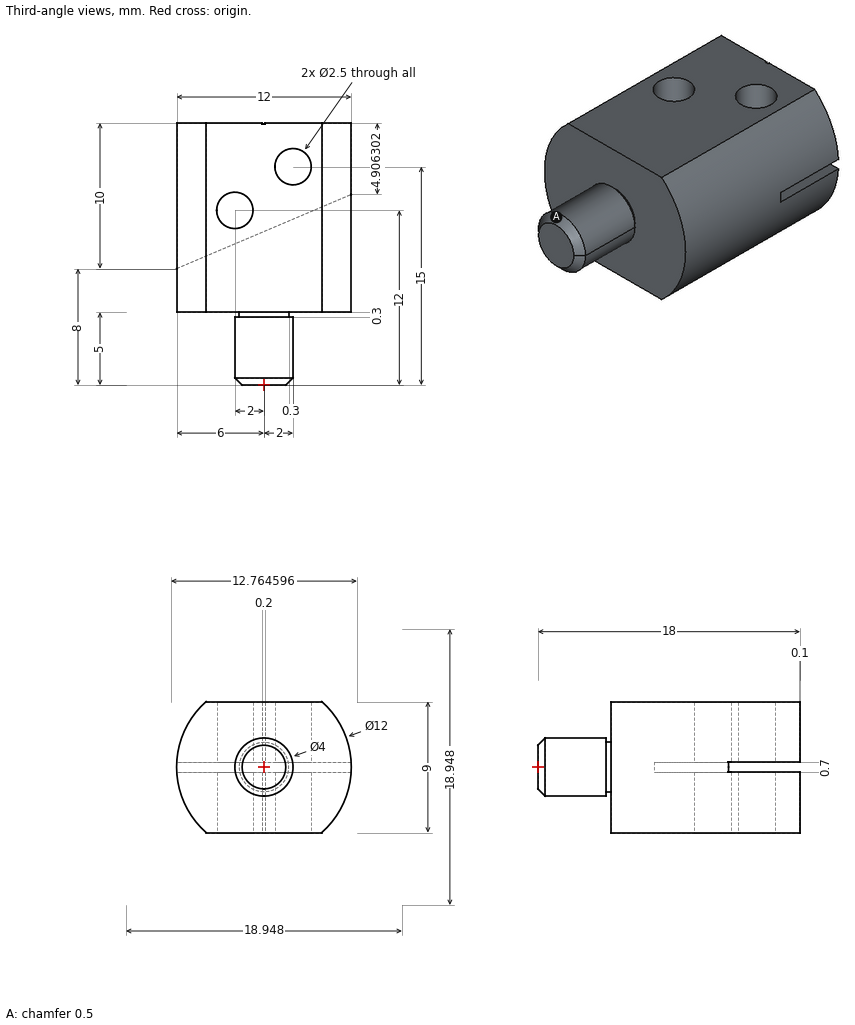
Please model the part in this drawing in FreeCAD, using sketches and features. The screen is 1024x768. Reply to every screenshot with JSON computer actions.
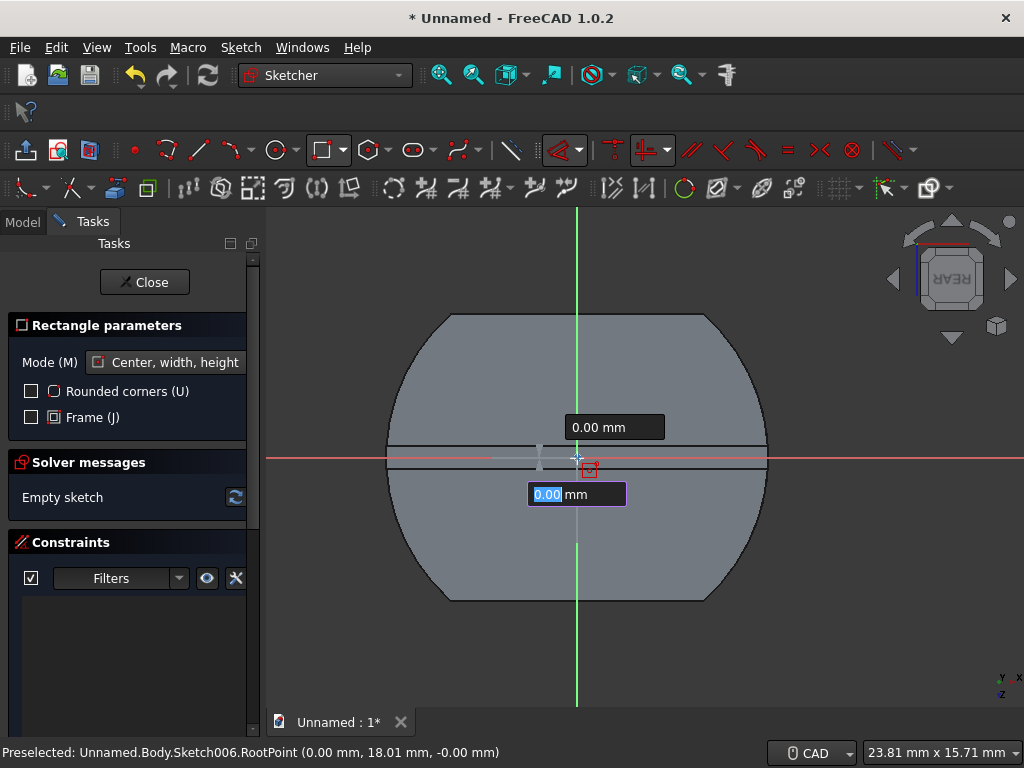
{"action": "scroll", "coordinate": [580, 314], "scroll_direction": "up", "scroll_amount": 9}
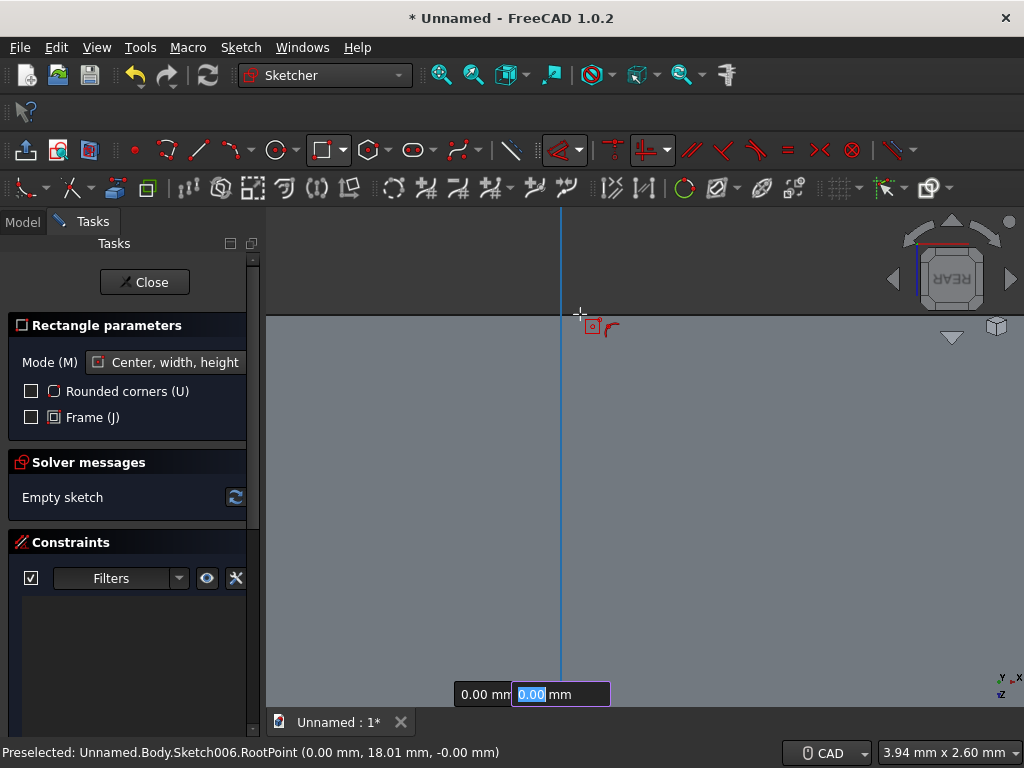
{"action": "left_click", "coordinate": [580, 315]}
{"action": "key", "text": "Escape"}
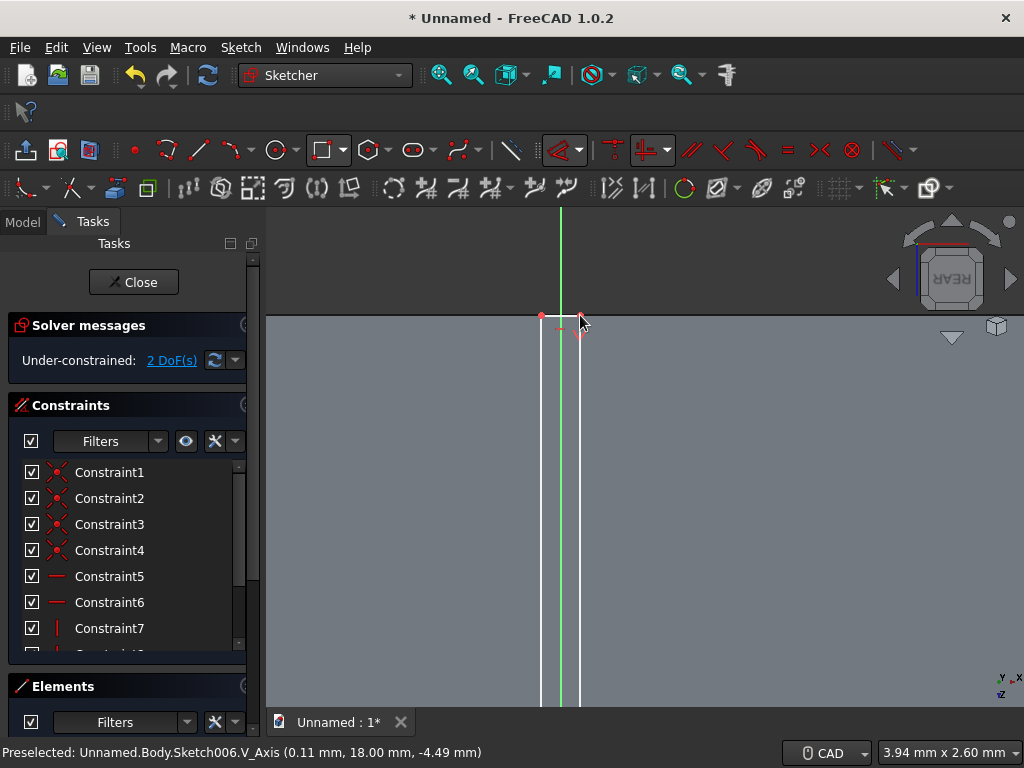
{"action": "left_click", "coordinate": [580, 662]}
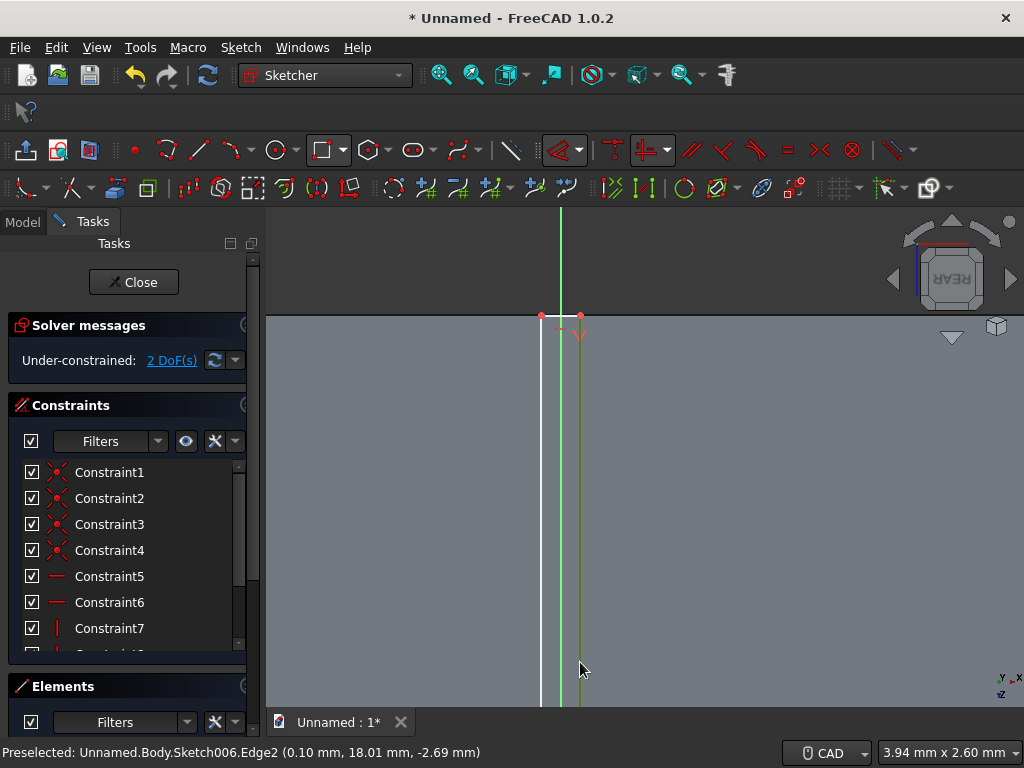
{"action": "left_click", "coordinate": [582, 150]}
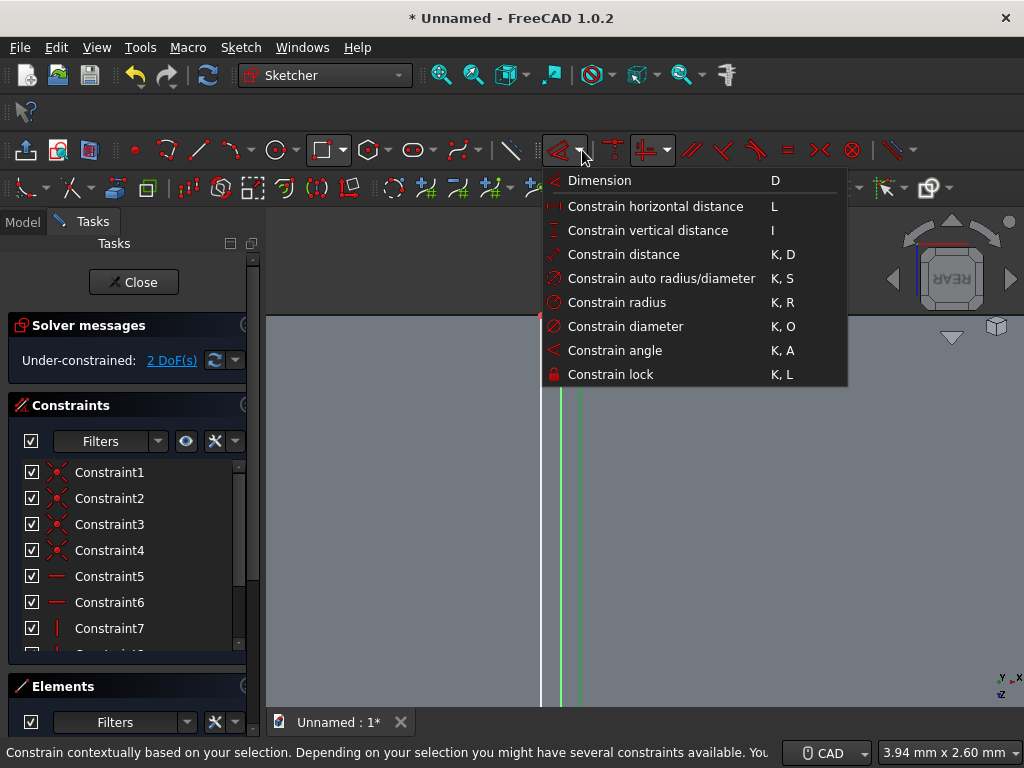
{"action": "left_click", "coordinate": [695, 230]}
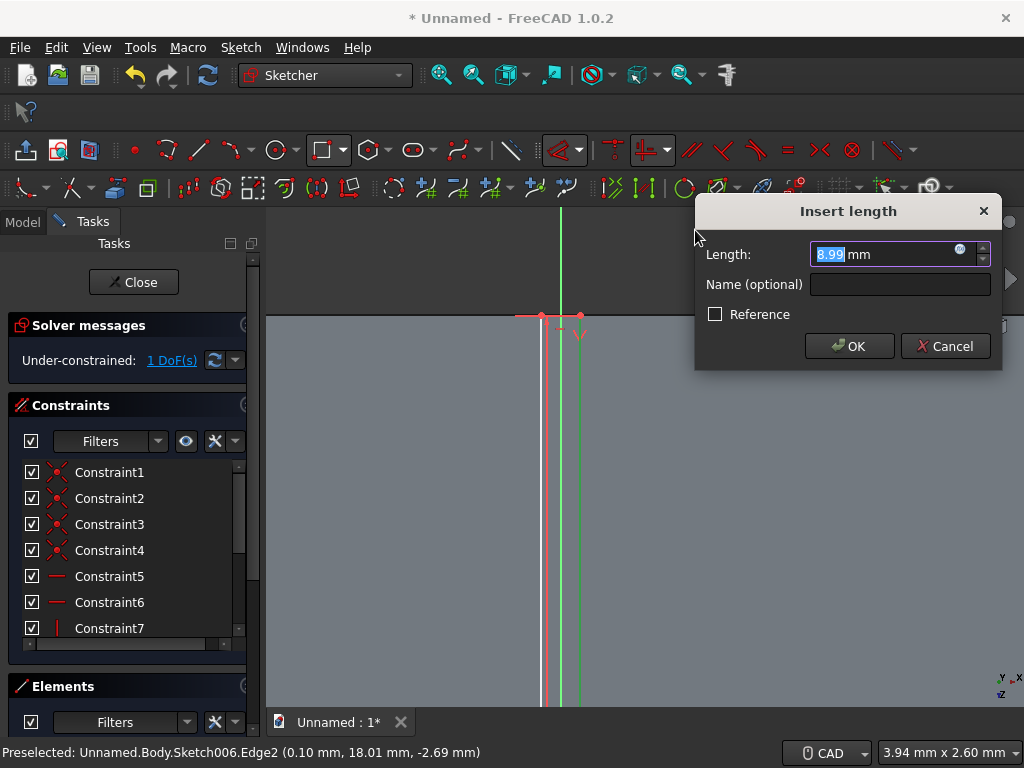
{"action": "type", "text": "9"}
{"action": "key", "text": "Return"}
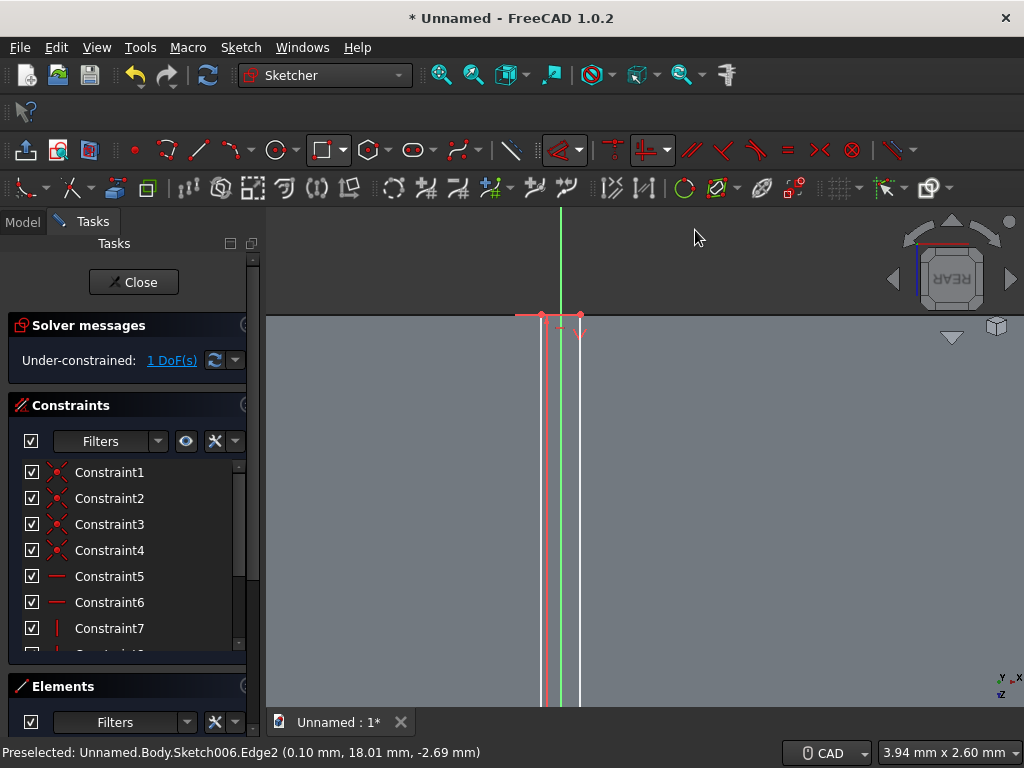
{"action": "scroll", "coordinate": [580, 314], "scroll_direction": "down", "scroll_amount": 9}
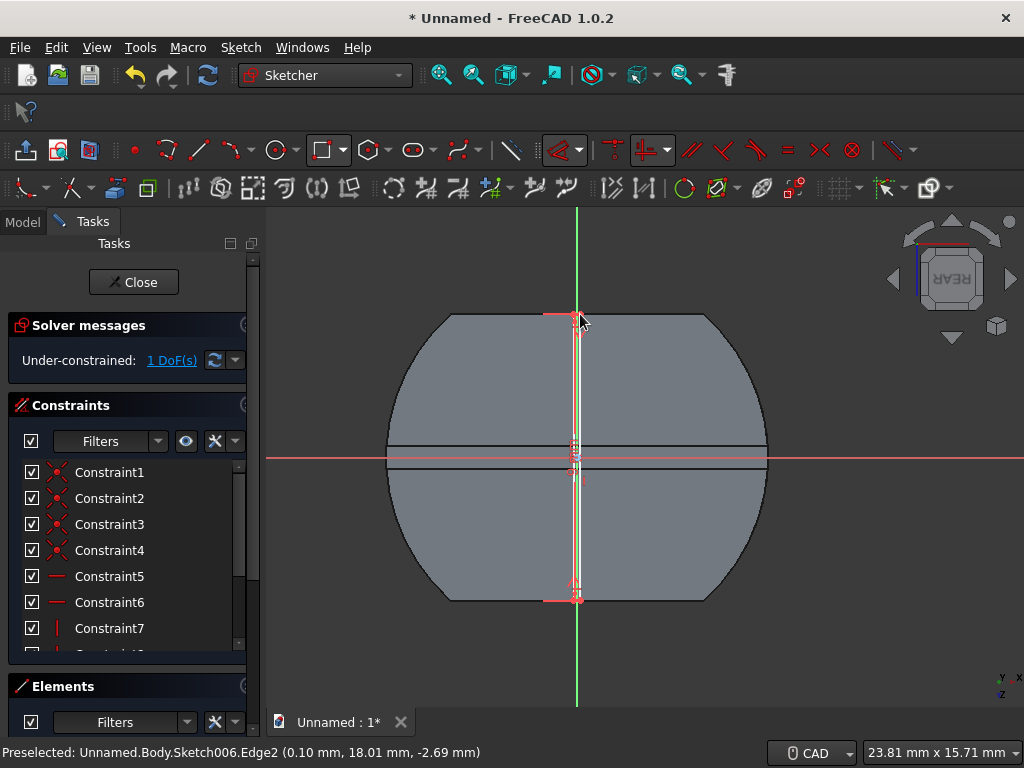
{"action": "scroll", "coordinate": [576, 601], "scroll_direction": "up", "scroll_amount": 10}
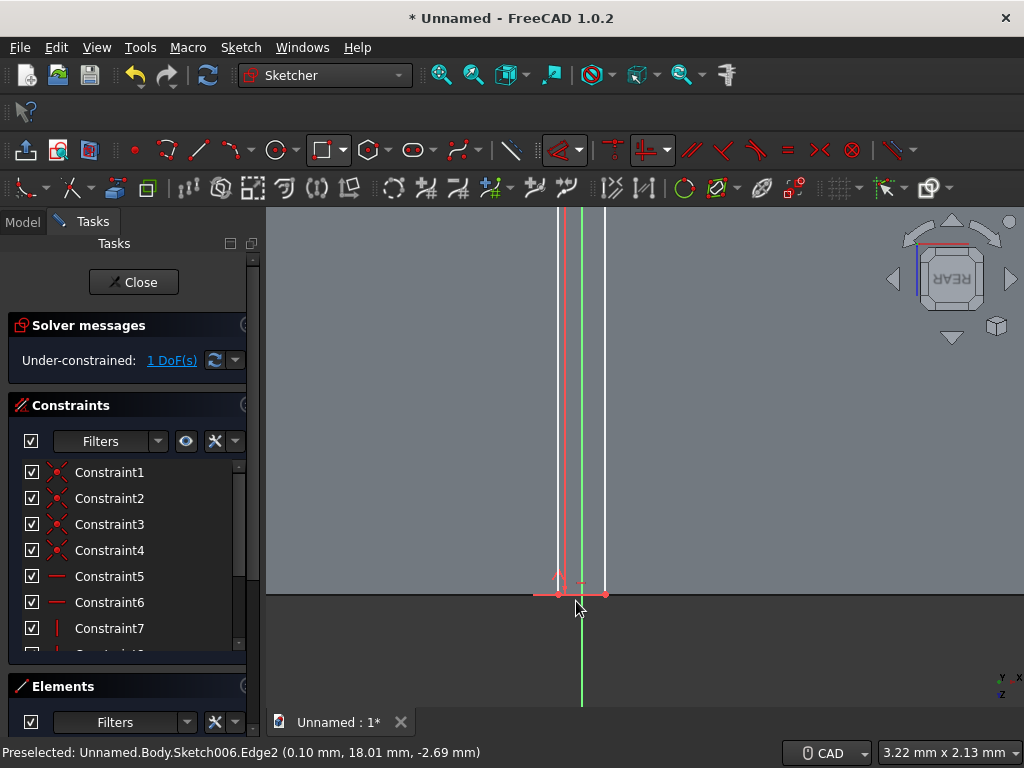
{"action": "left_click", "coordinate": [577, 595]}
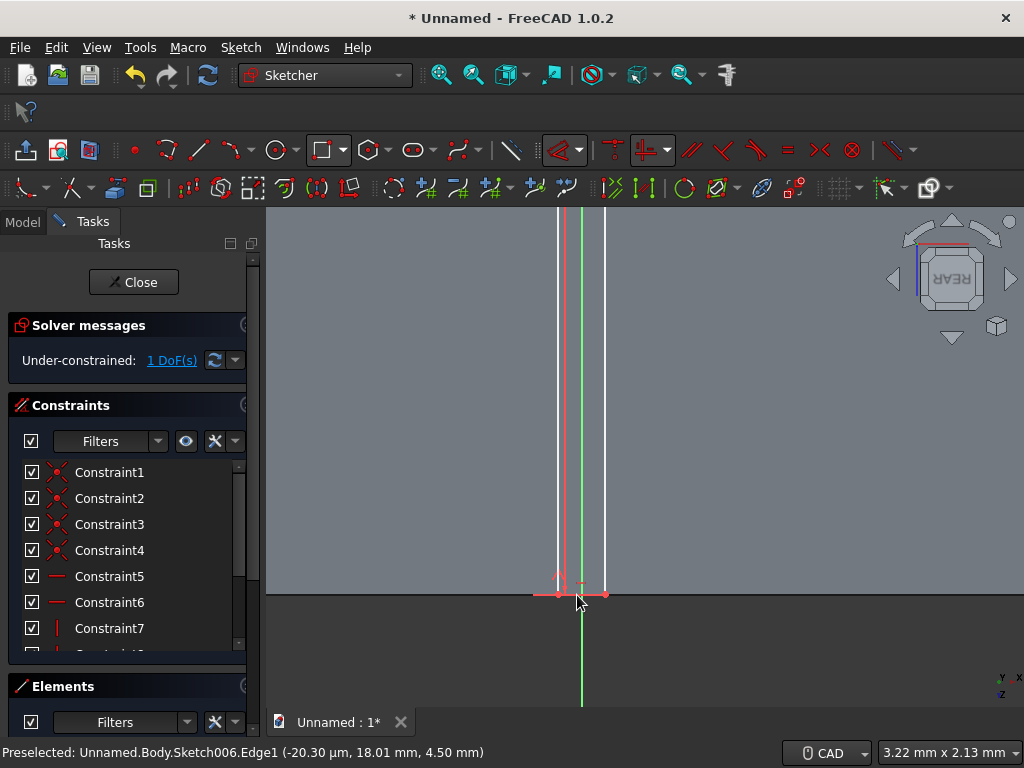
{"action": "key", "text": "l"}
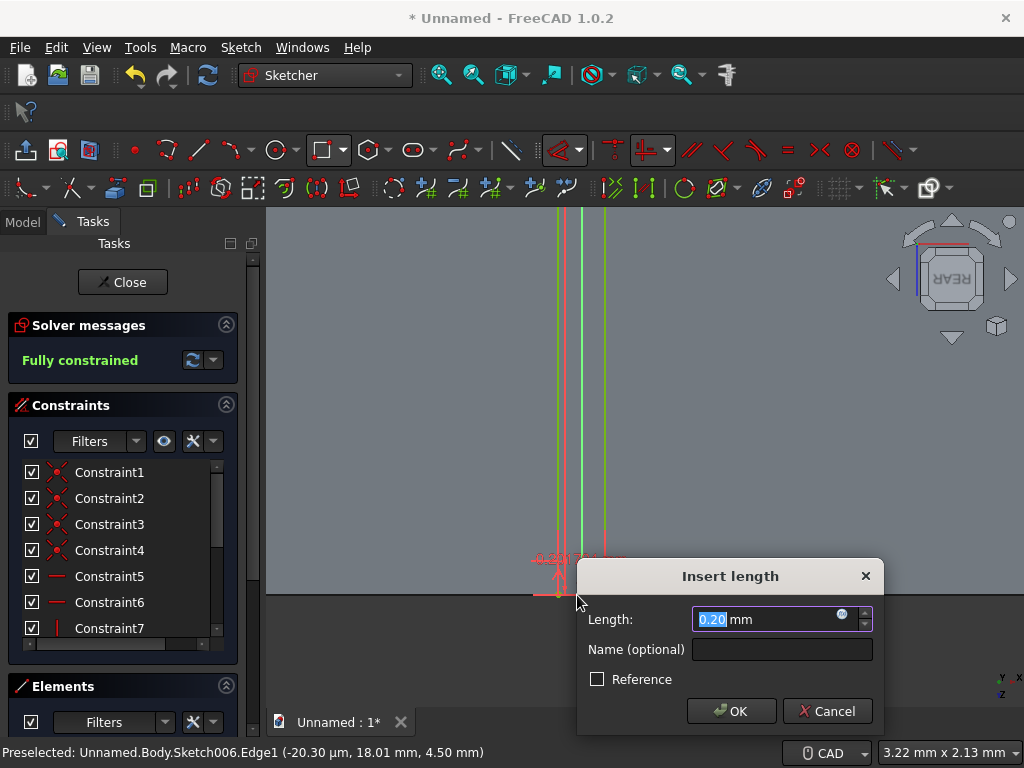
{"action": "type", "text": "0.2"}
{"action": "key", "text": "Return"}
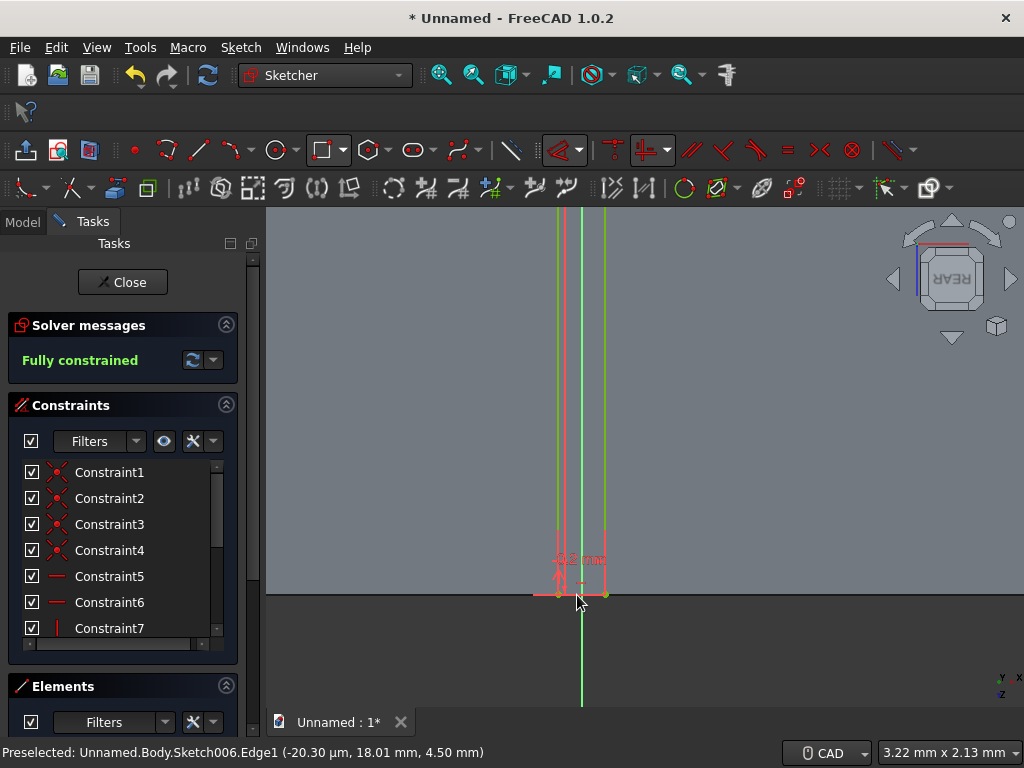
{"action": "left_click", "coordinate": [123, 282]}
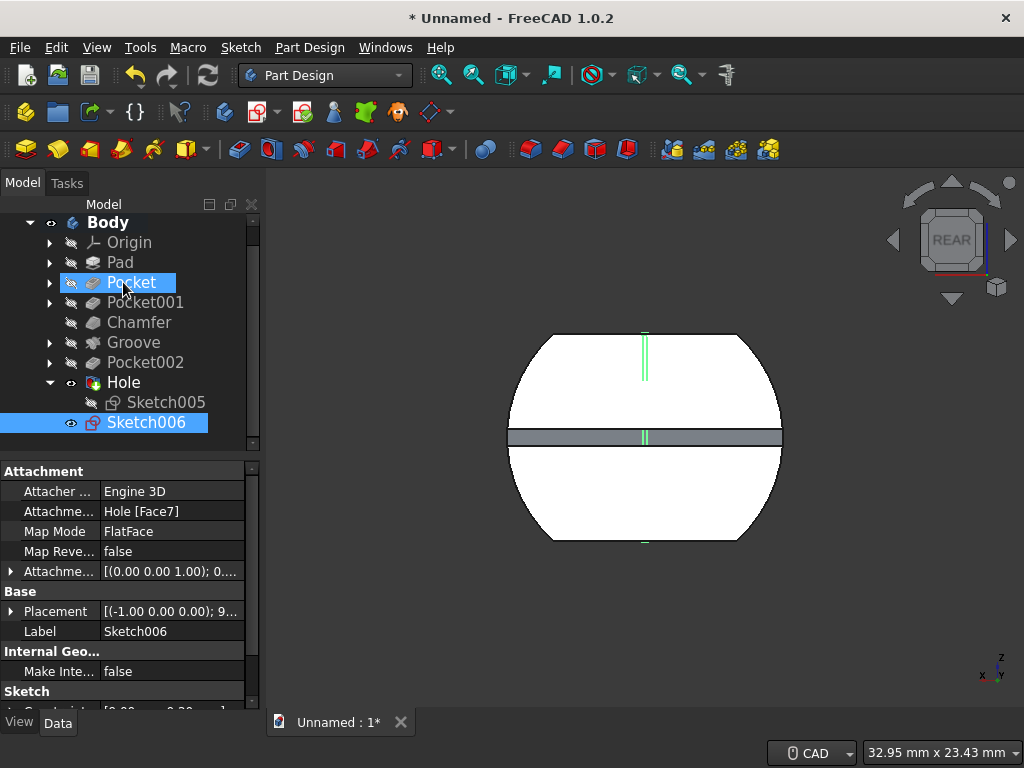
{"action": "left_click", "coordinate": [240, 150]}